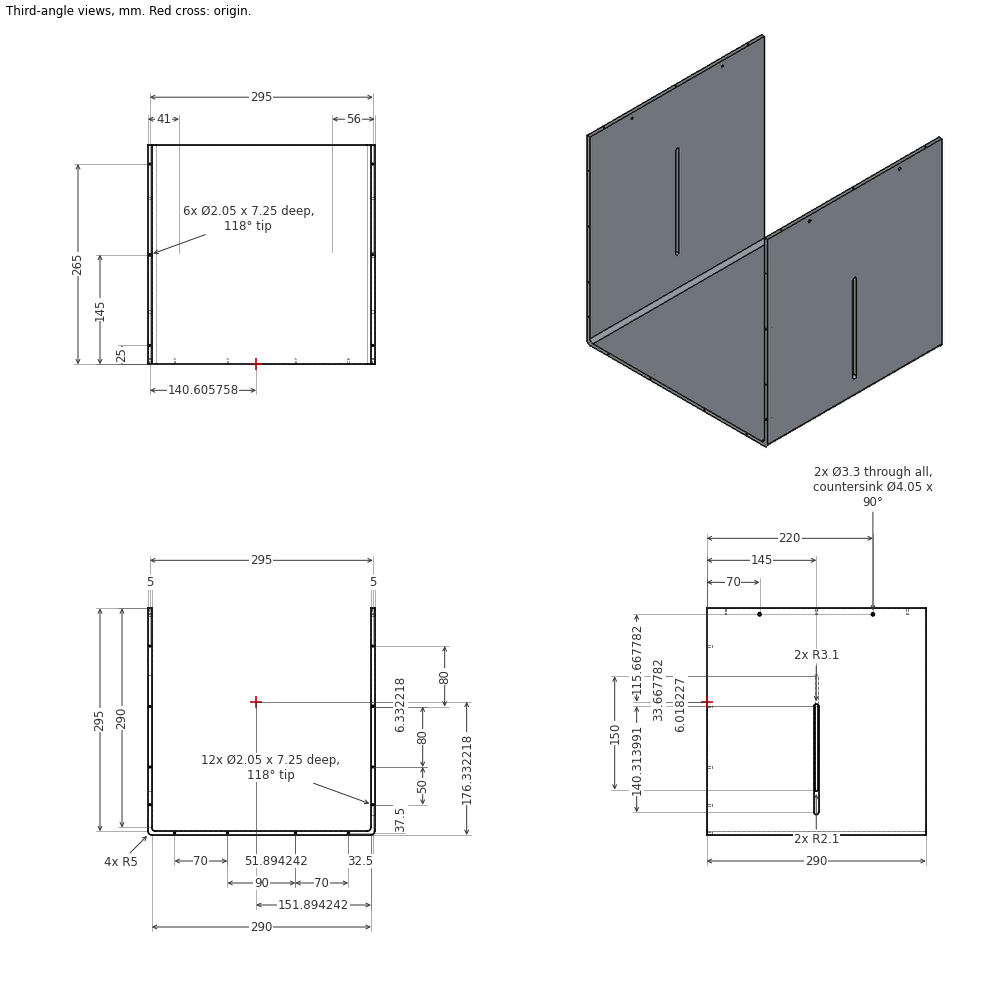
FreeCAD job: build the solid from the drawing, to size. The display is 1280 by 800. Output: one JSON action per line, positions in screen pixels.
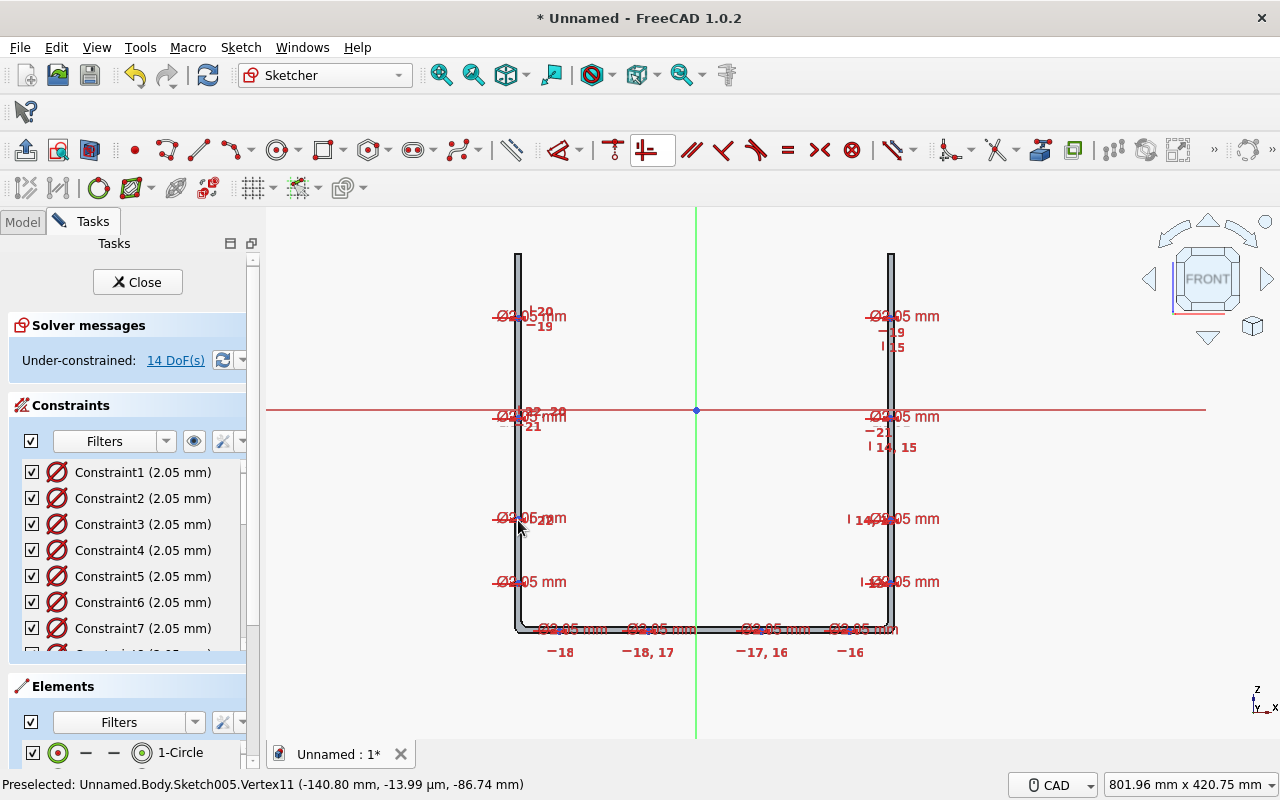
{"action": "left_click", "coordinate": [518, 520]}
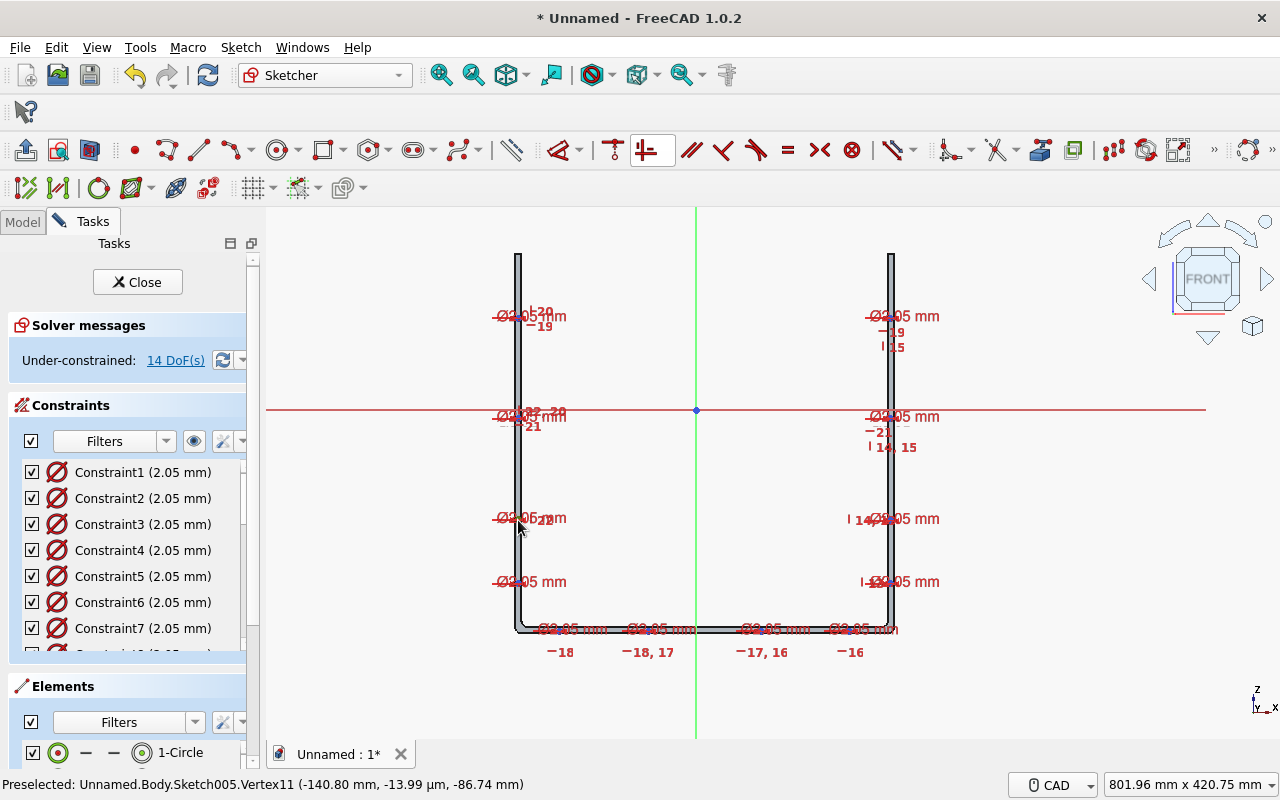
{"action": "left_click", "coordinate": [518, 584]}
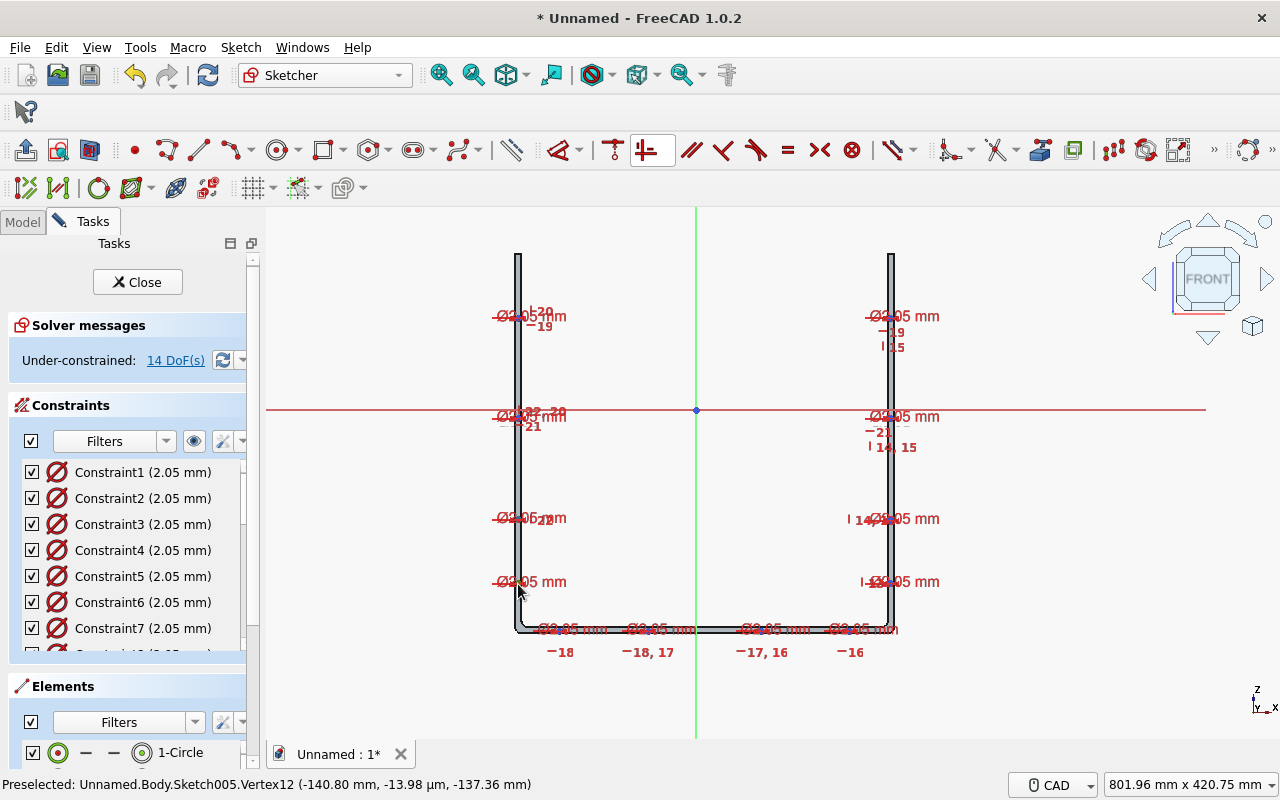
{"action": "left_click", "coordinate": [670, 150]}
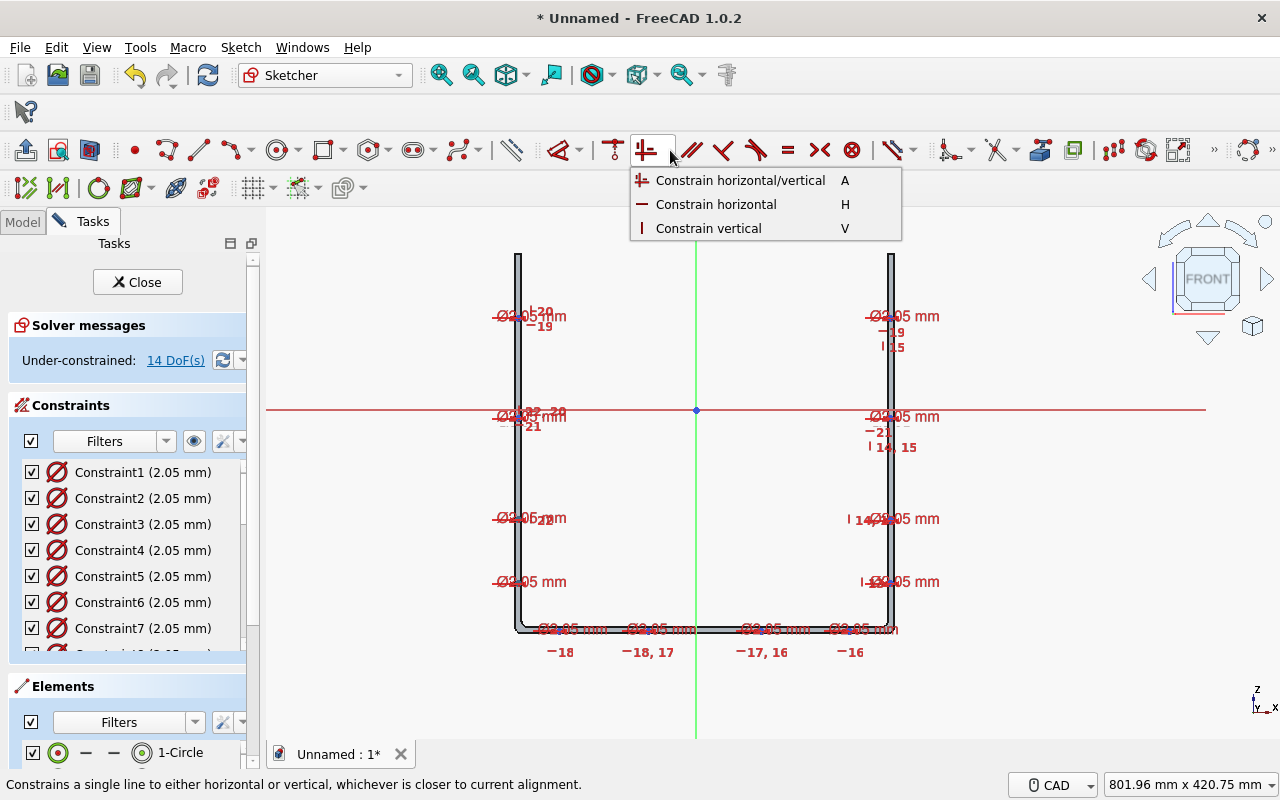
{"action": "left_click", "coordinate": [766, 228]}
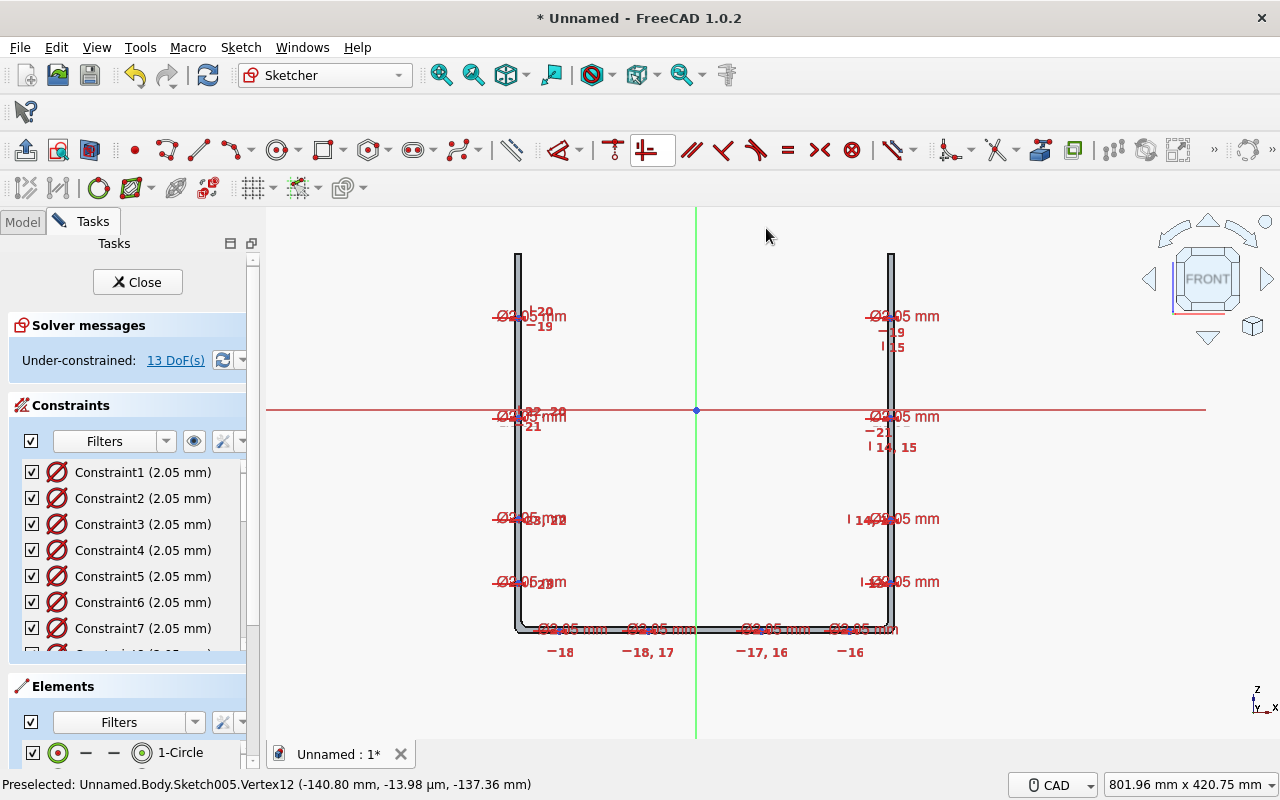
{"action": "left_click", "coordinate": [558, 150]}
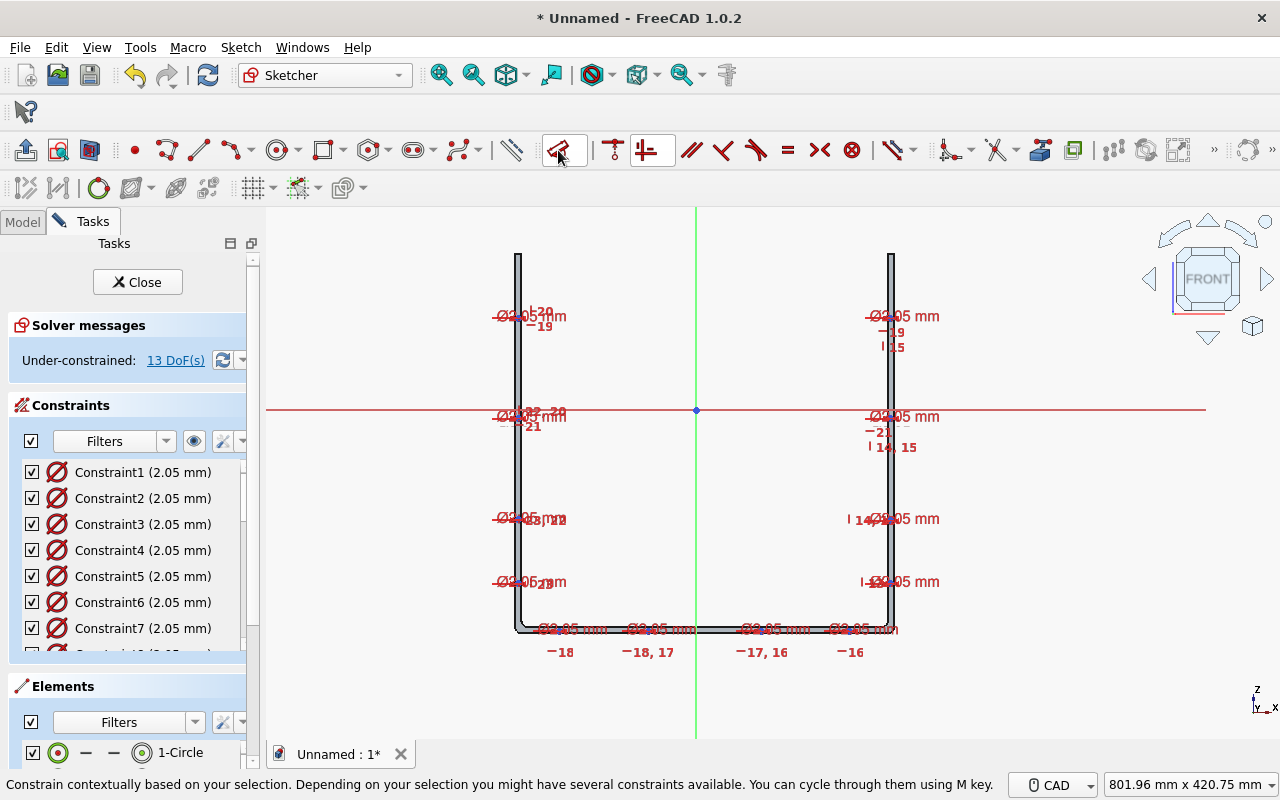
{"action": "left_click", "coordinate": [891, 584]}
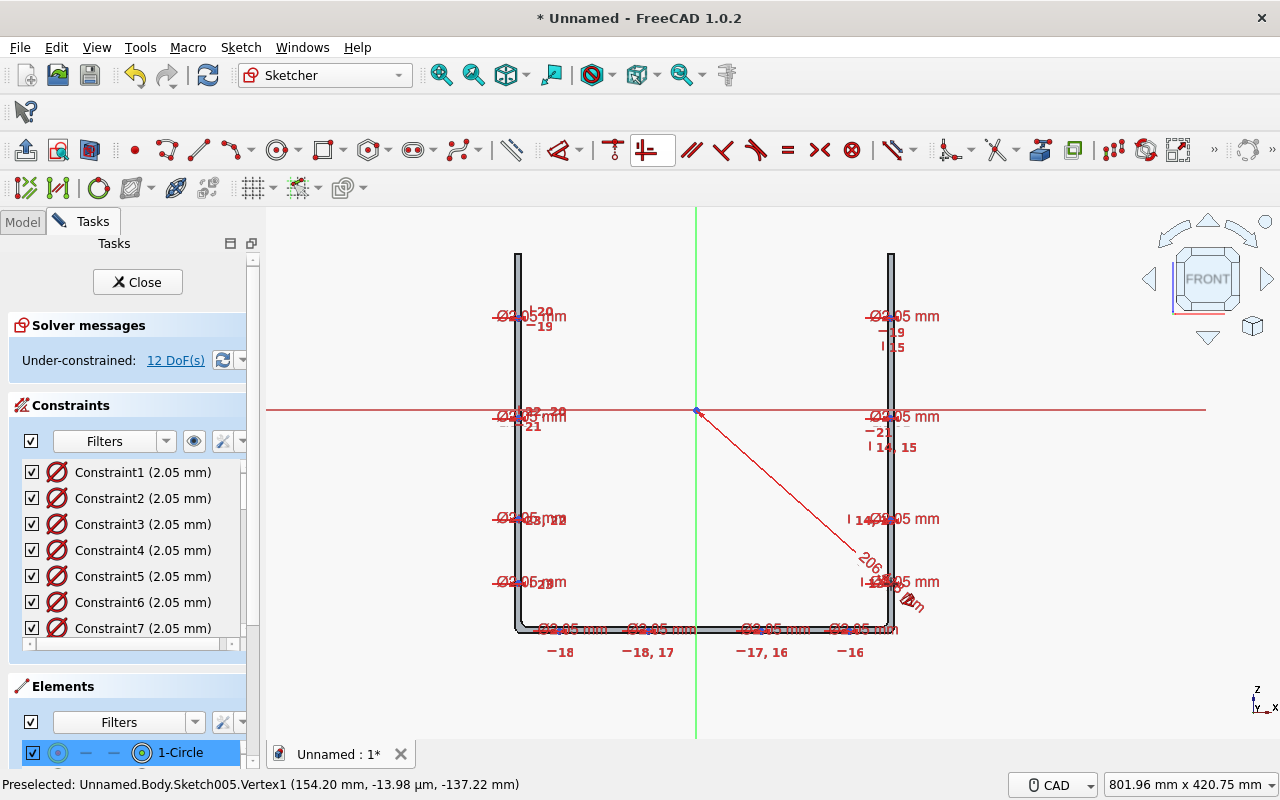
{"action": "left_click", "coordinate": [891, 521]}
{"action": "left_click", "coordinate": [925, 552]}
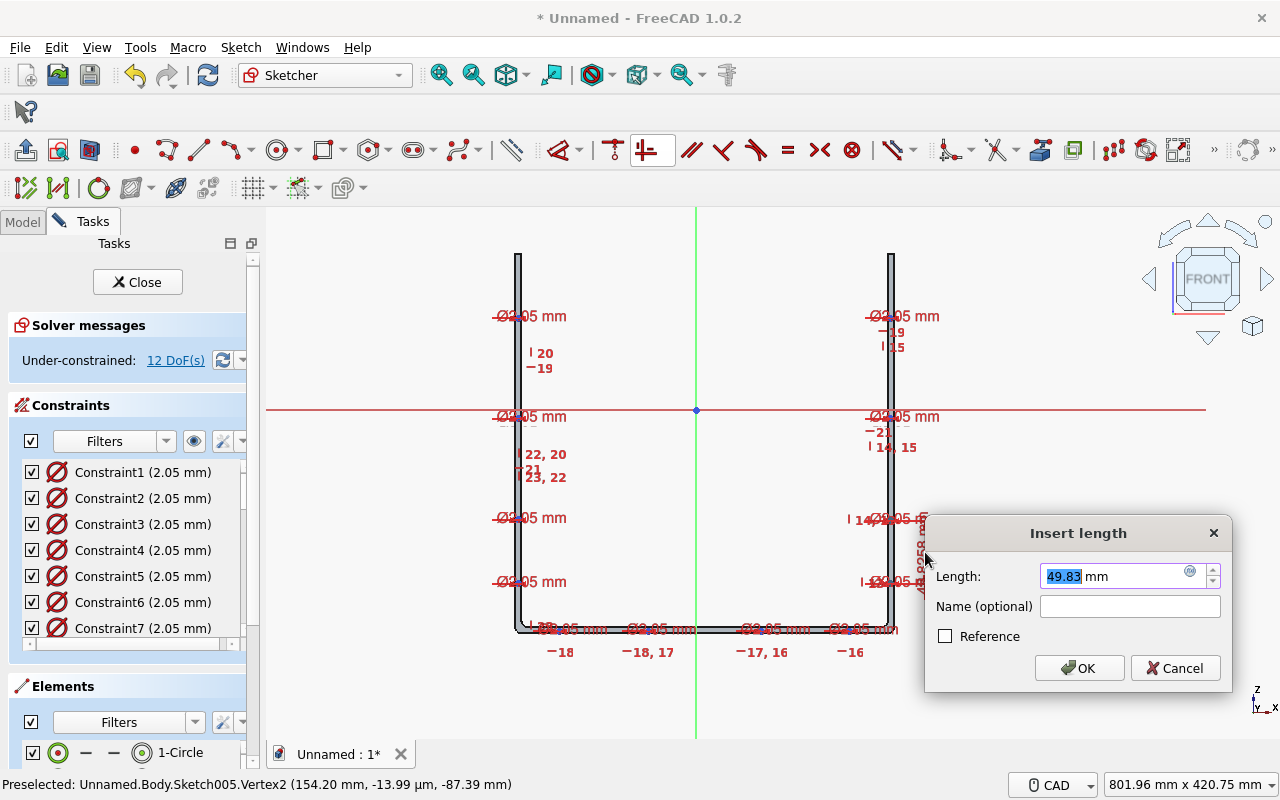
{"action": "type", "text": "50"}
{"action": "key", "text": "Return"}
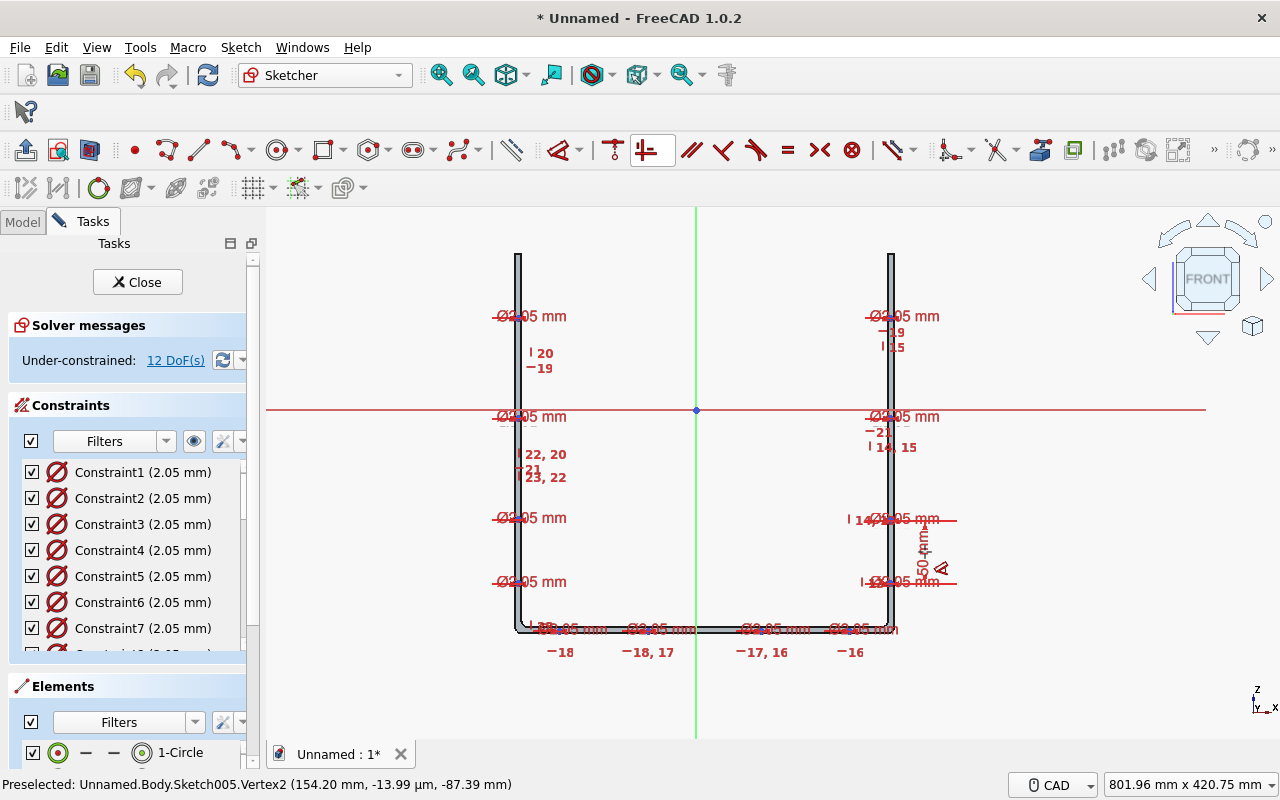
{"action": "left_click", "coordinate": [891, 521]}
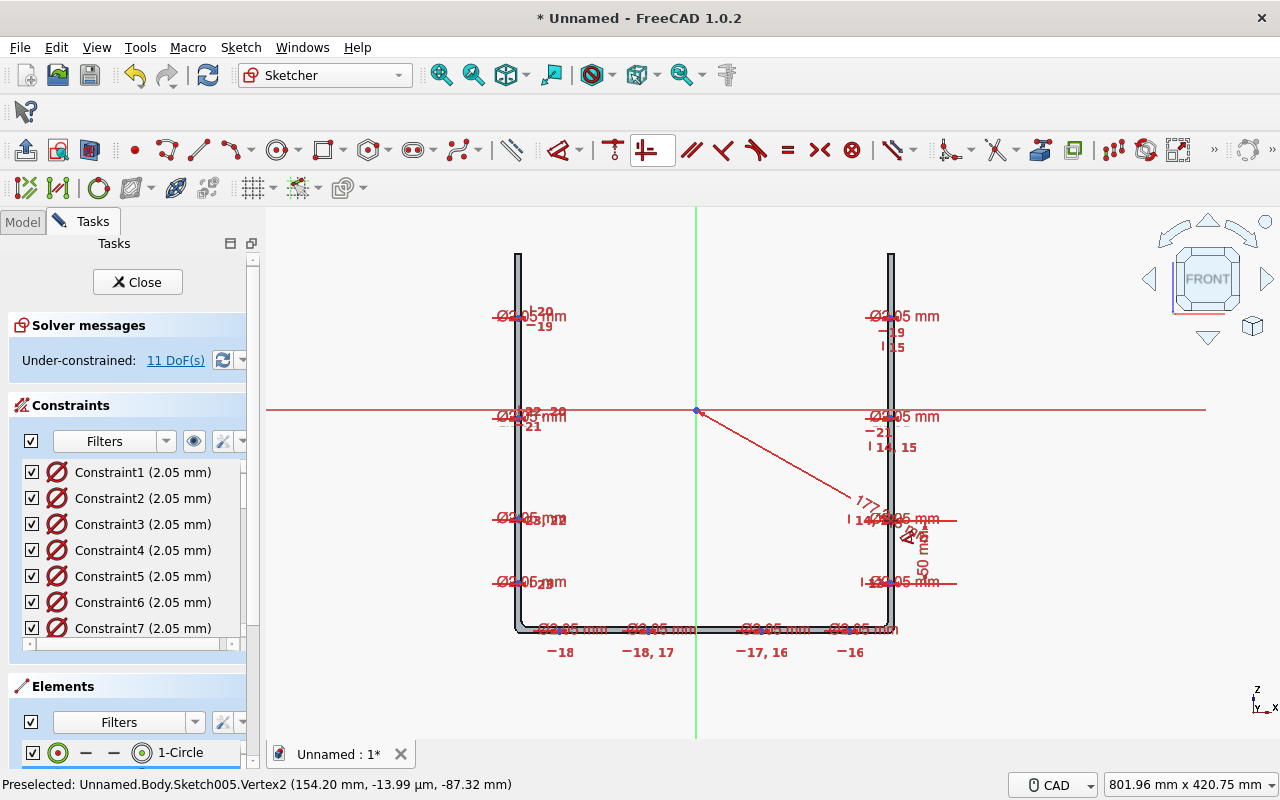
{"action": "left_click", "coordinate": [891, 419]}
{"action": "left_click", "coordinate": [925, 470]}